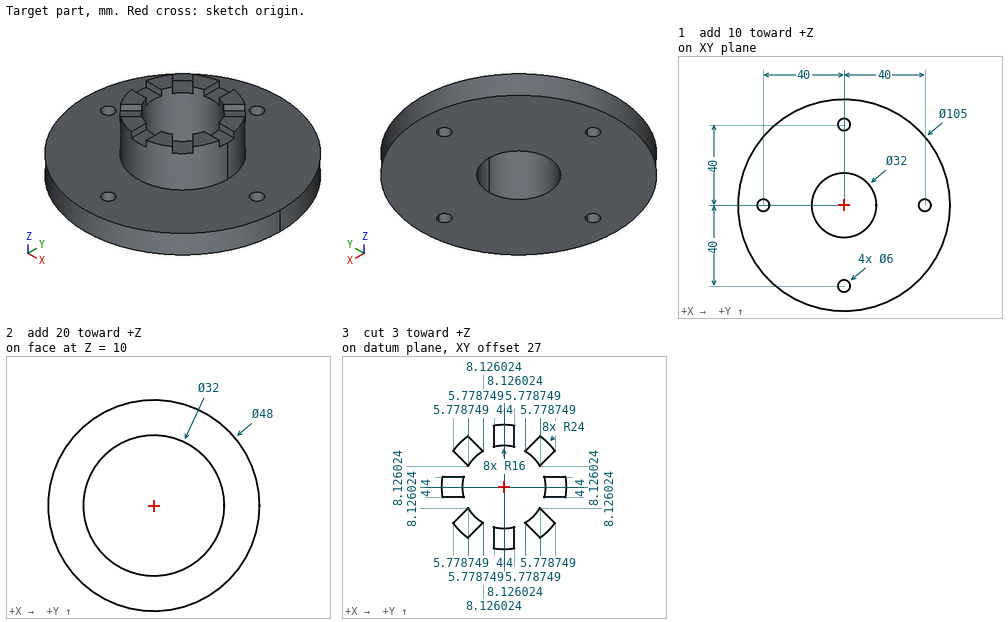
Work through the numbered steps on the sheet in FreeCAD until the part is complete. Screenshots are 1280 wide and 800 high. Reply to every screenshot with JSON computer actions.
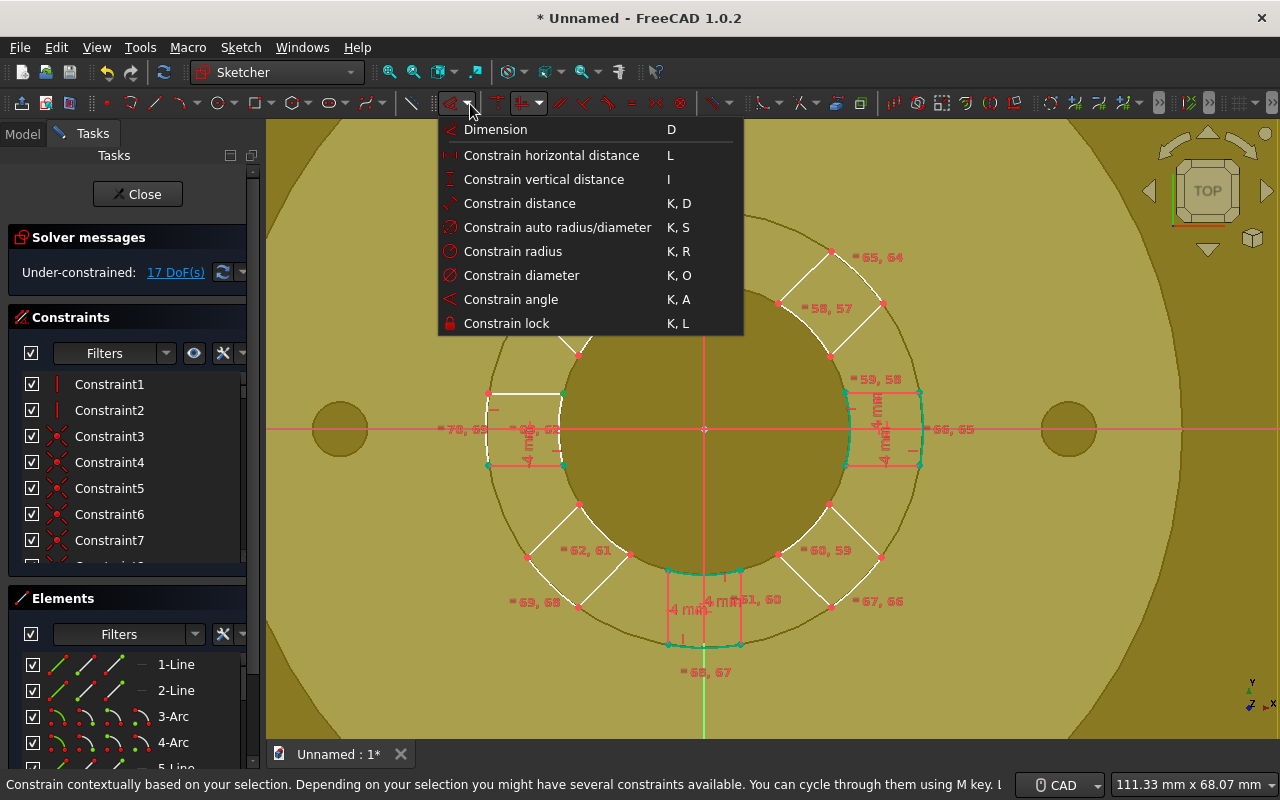
{"action": "left_click", "coordinate": [591, 179]}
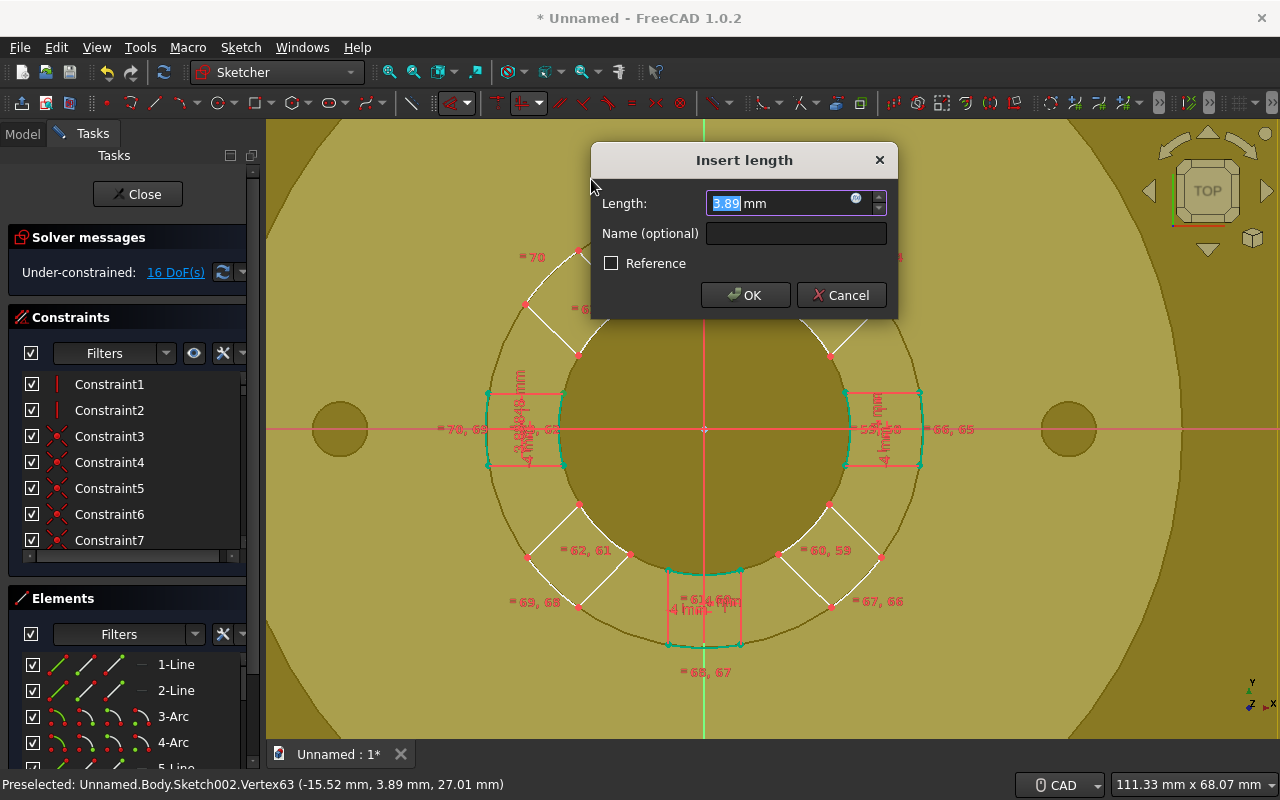
{"action": "type", "text": "4"}
{"action": "key", "text": "Return"}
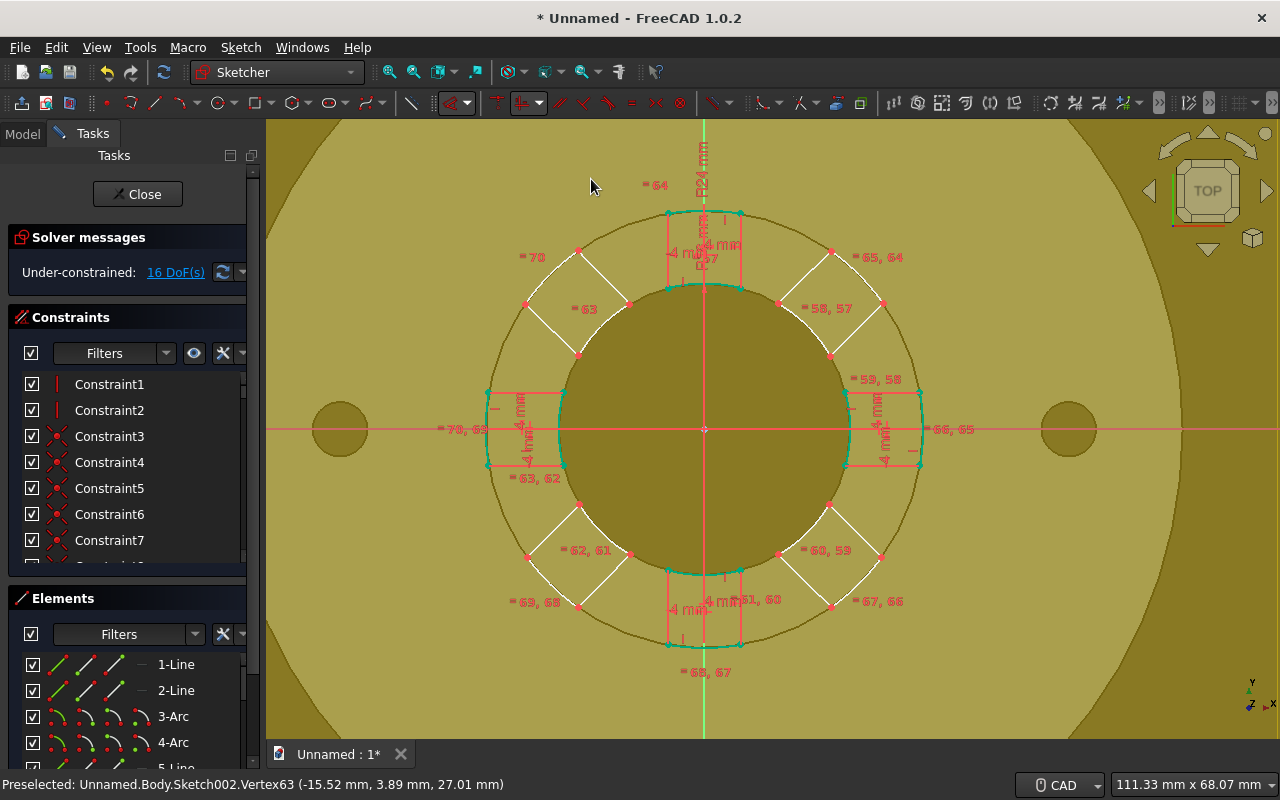
{"action": "left_click", "coordinate": [778, 304]}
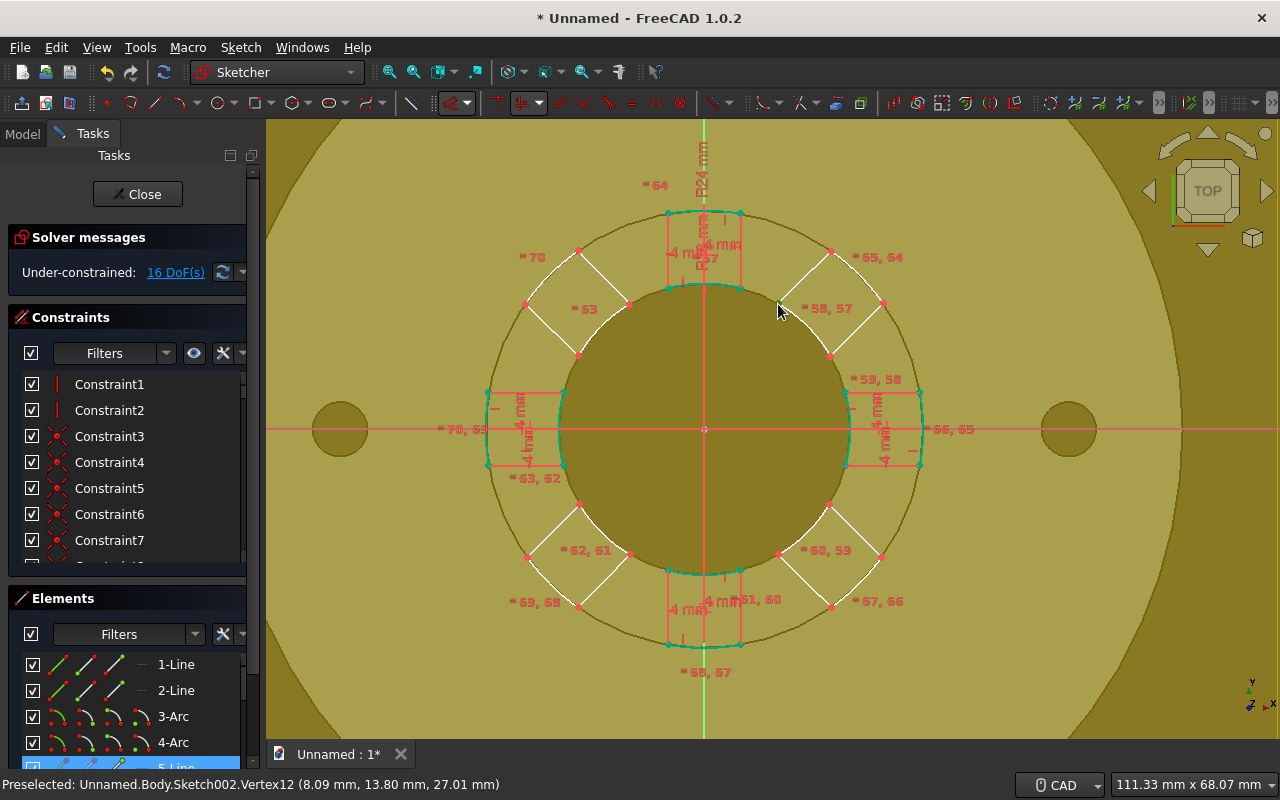
{"action": "left_click", "coordinate": [470, 104]}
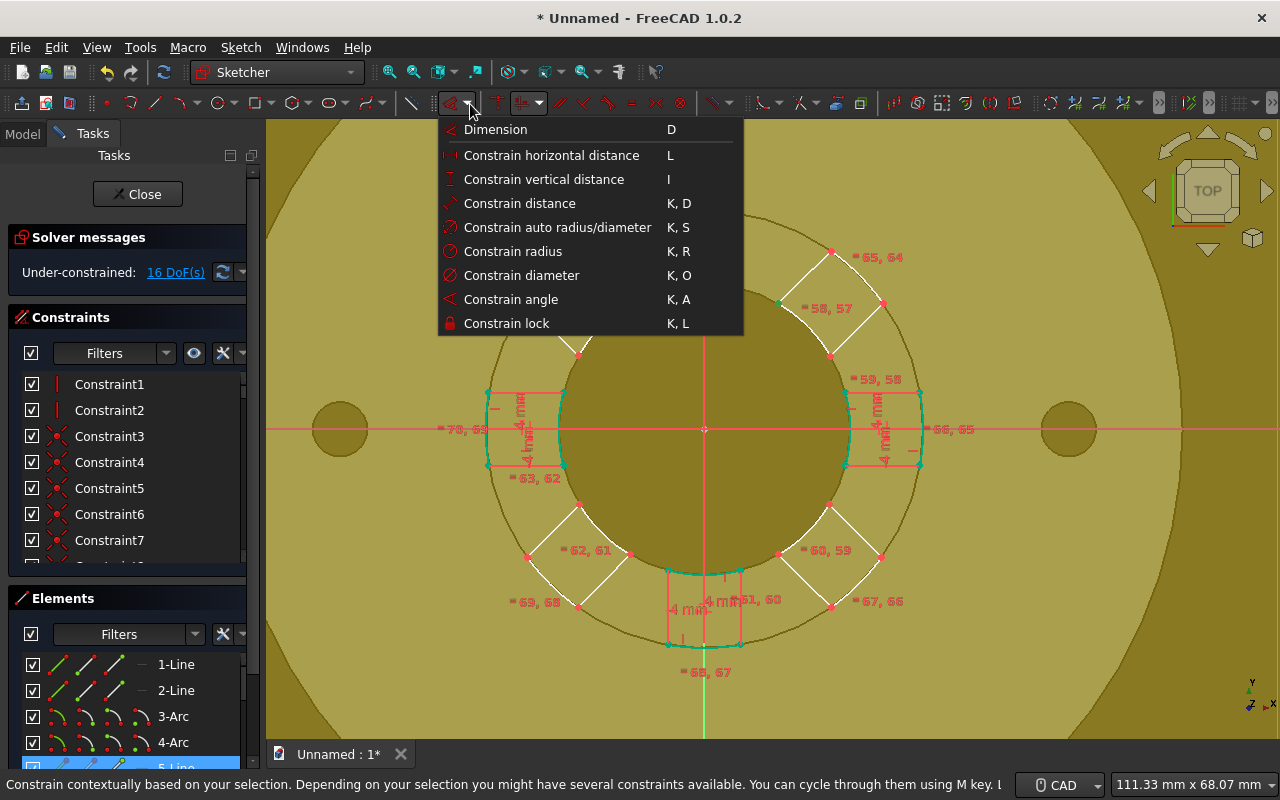
{"action": "left_click", "coordinate": [591, 155]}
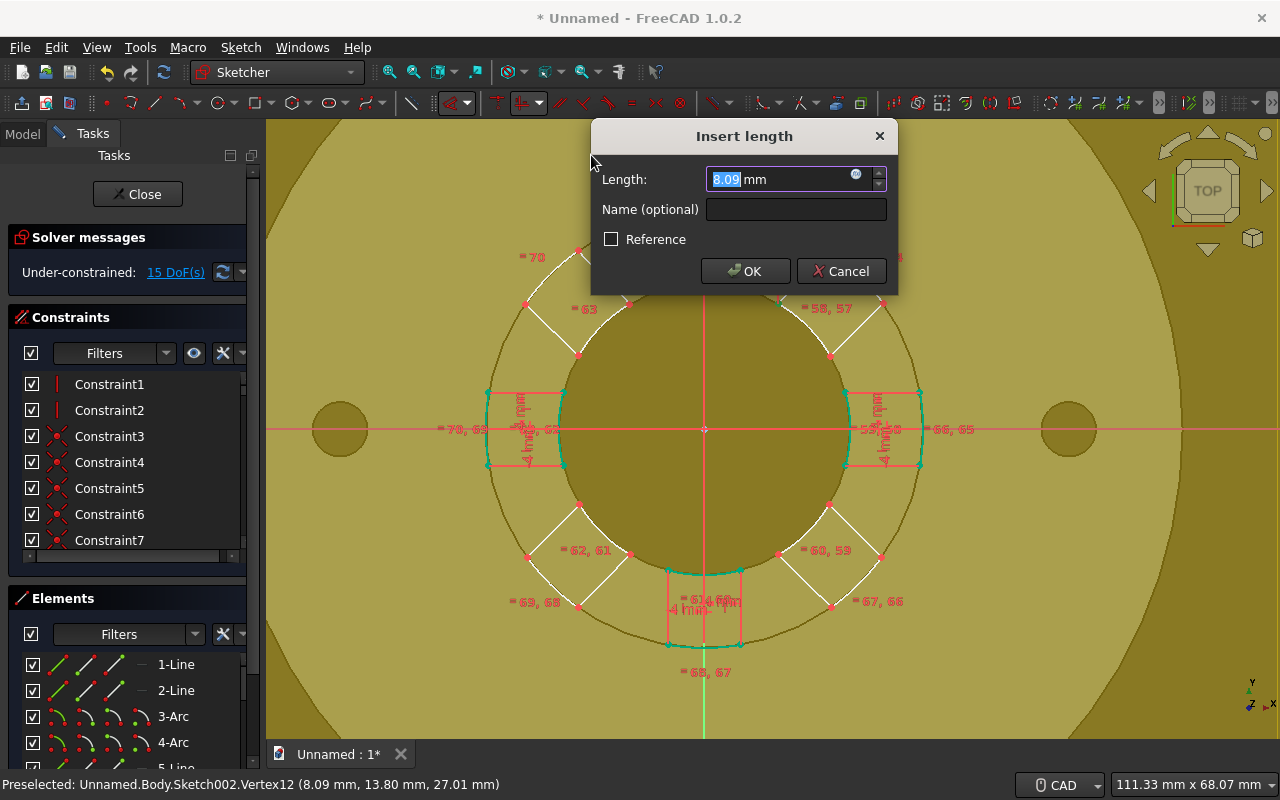
{"action": "type", "text": "8.126024"}
{"action": "key", "text": "Return"}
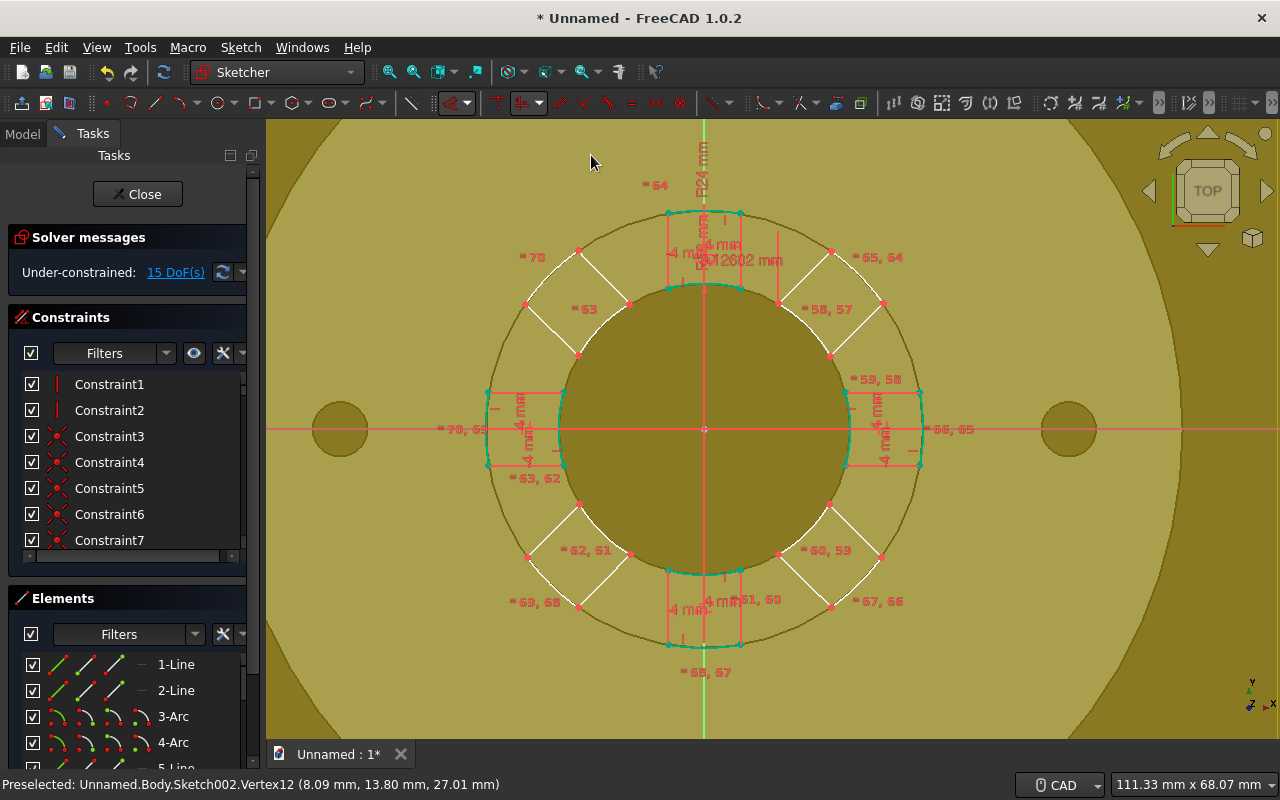
{"action": "left_click", "coordinate": [830, 356]}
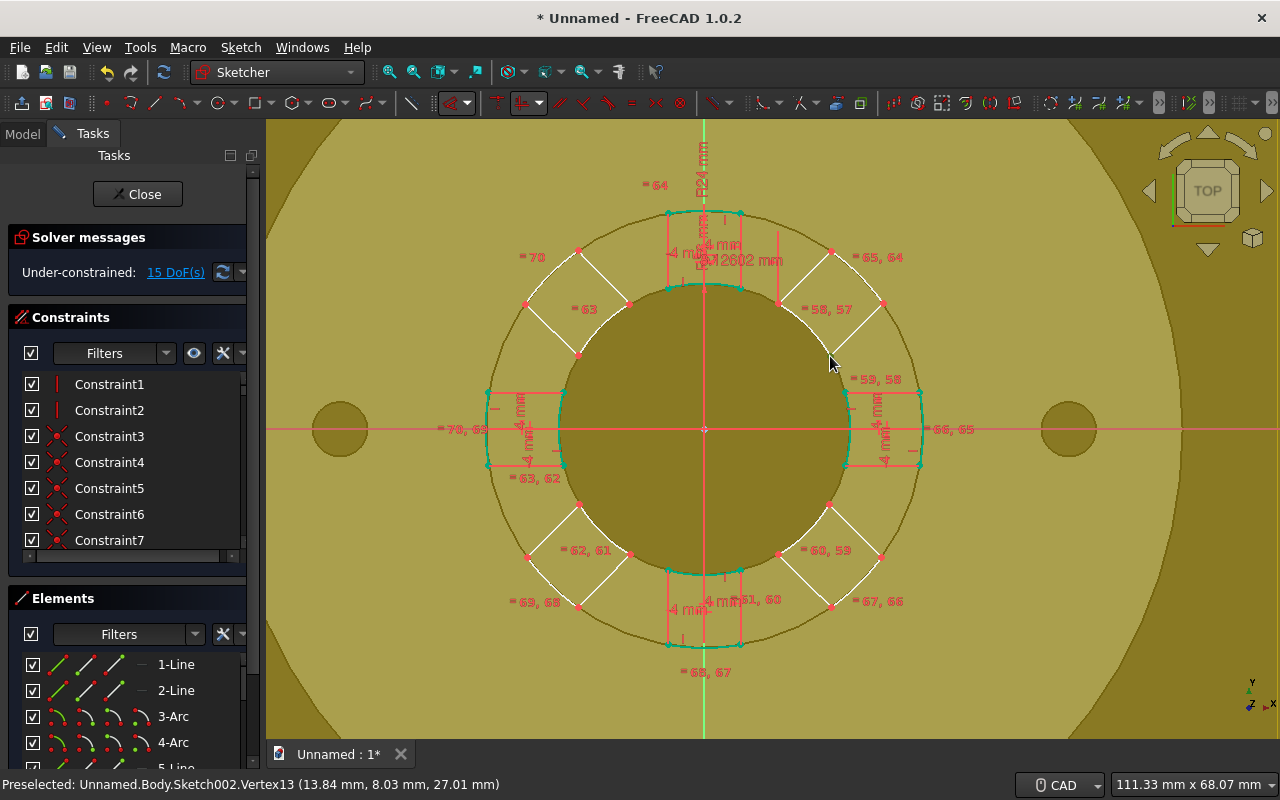
{"action": "left_click", "coordinate": [470, 104]}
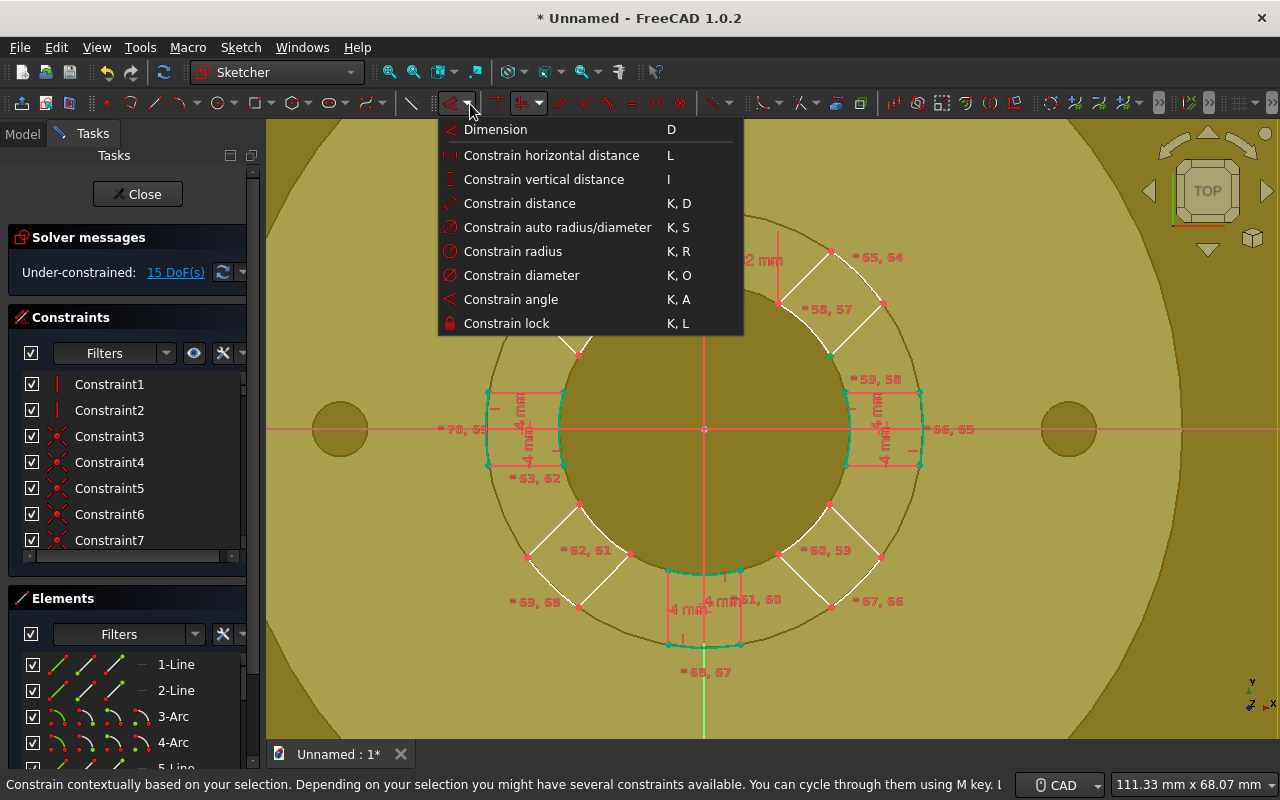
{"action": "left_click", "coordinate": [591, 179]}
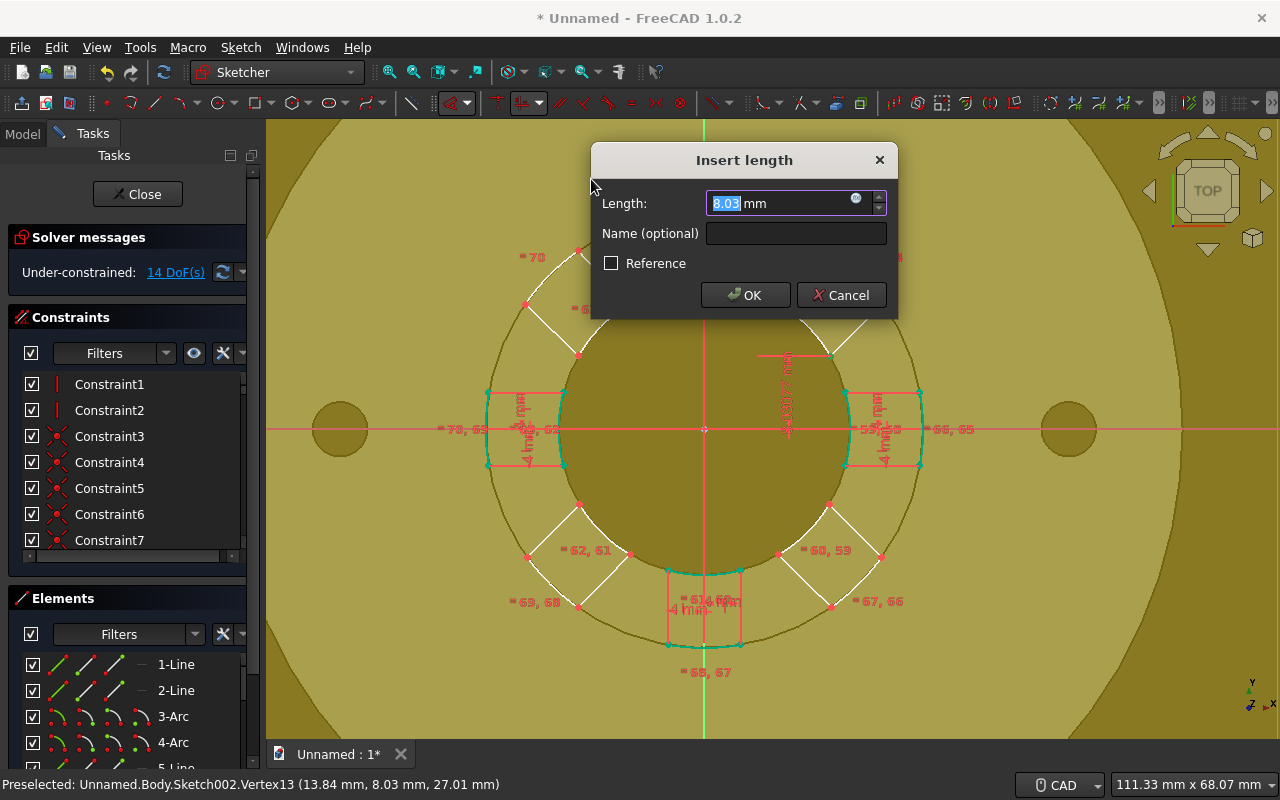
{"action": "type", "text": "8.126024"}
{"action": "key", "text": "Return"}